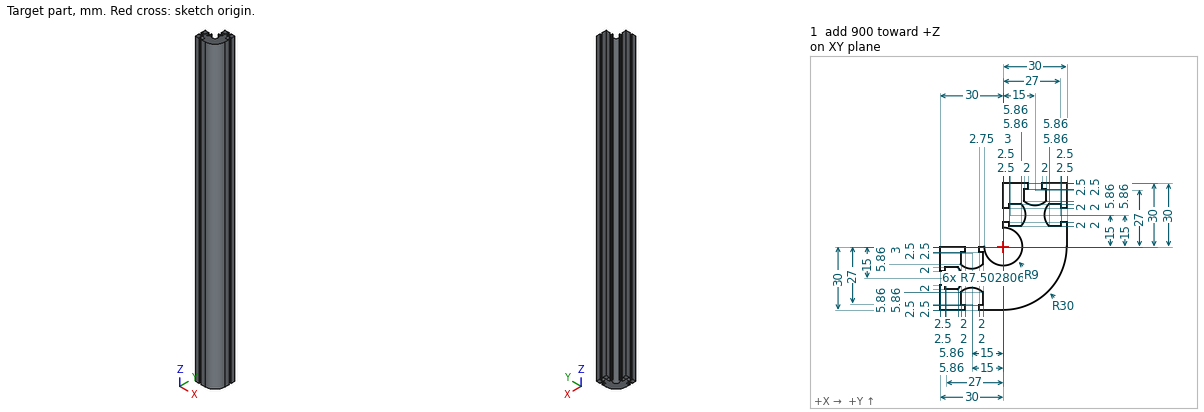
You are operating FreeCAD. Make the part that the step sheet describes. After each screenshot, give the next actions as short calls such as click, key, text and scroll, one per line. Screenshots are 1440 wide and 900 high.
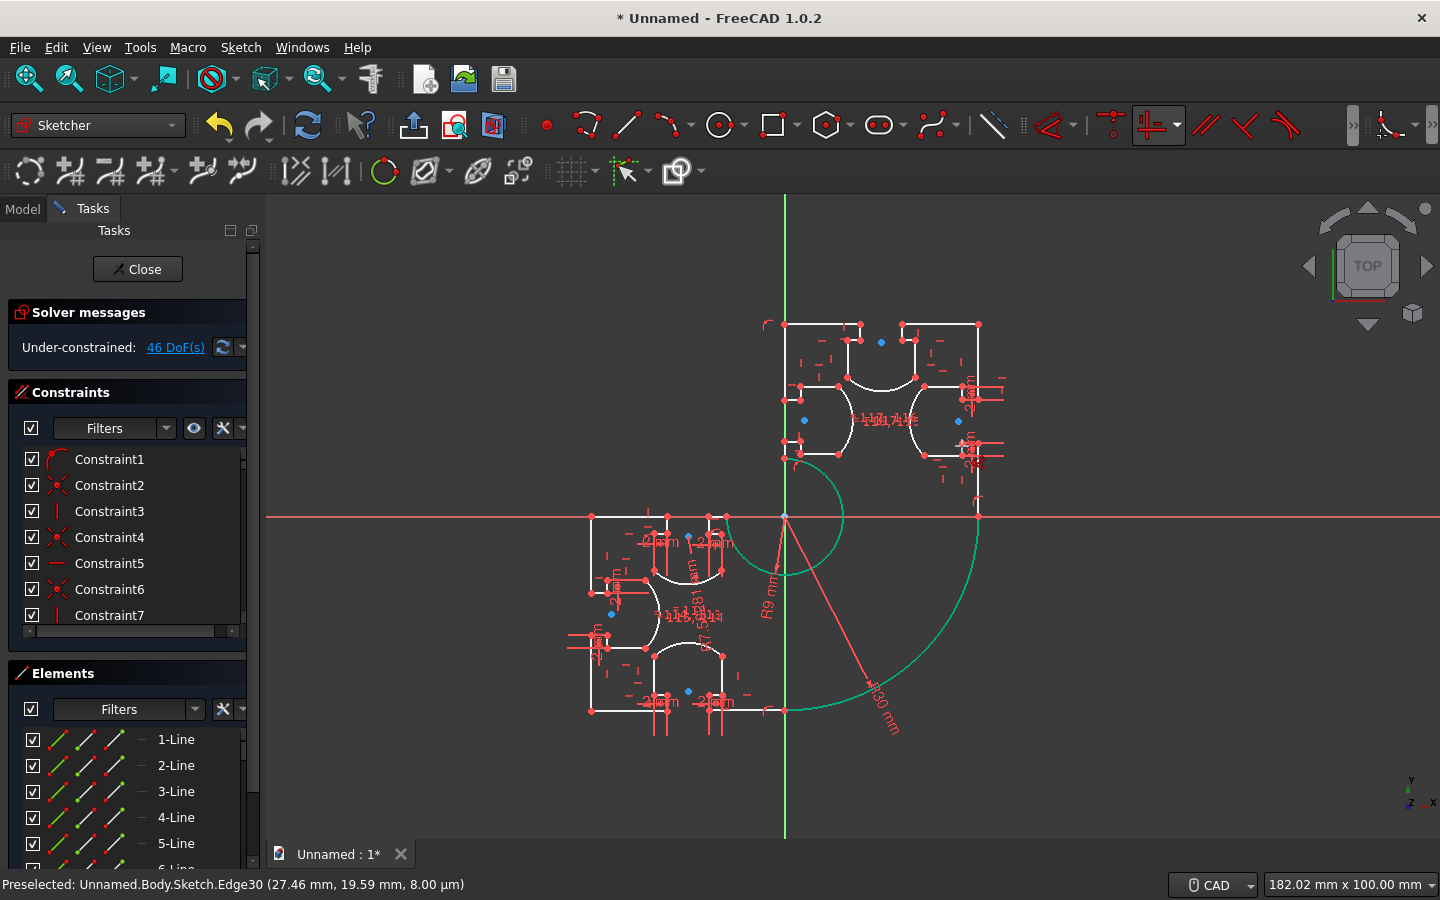
scroll(906, 340, up, 7)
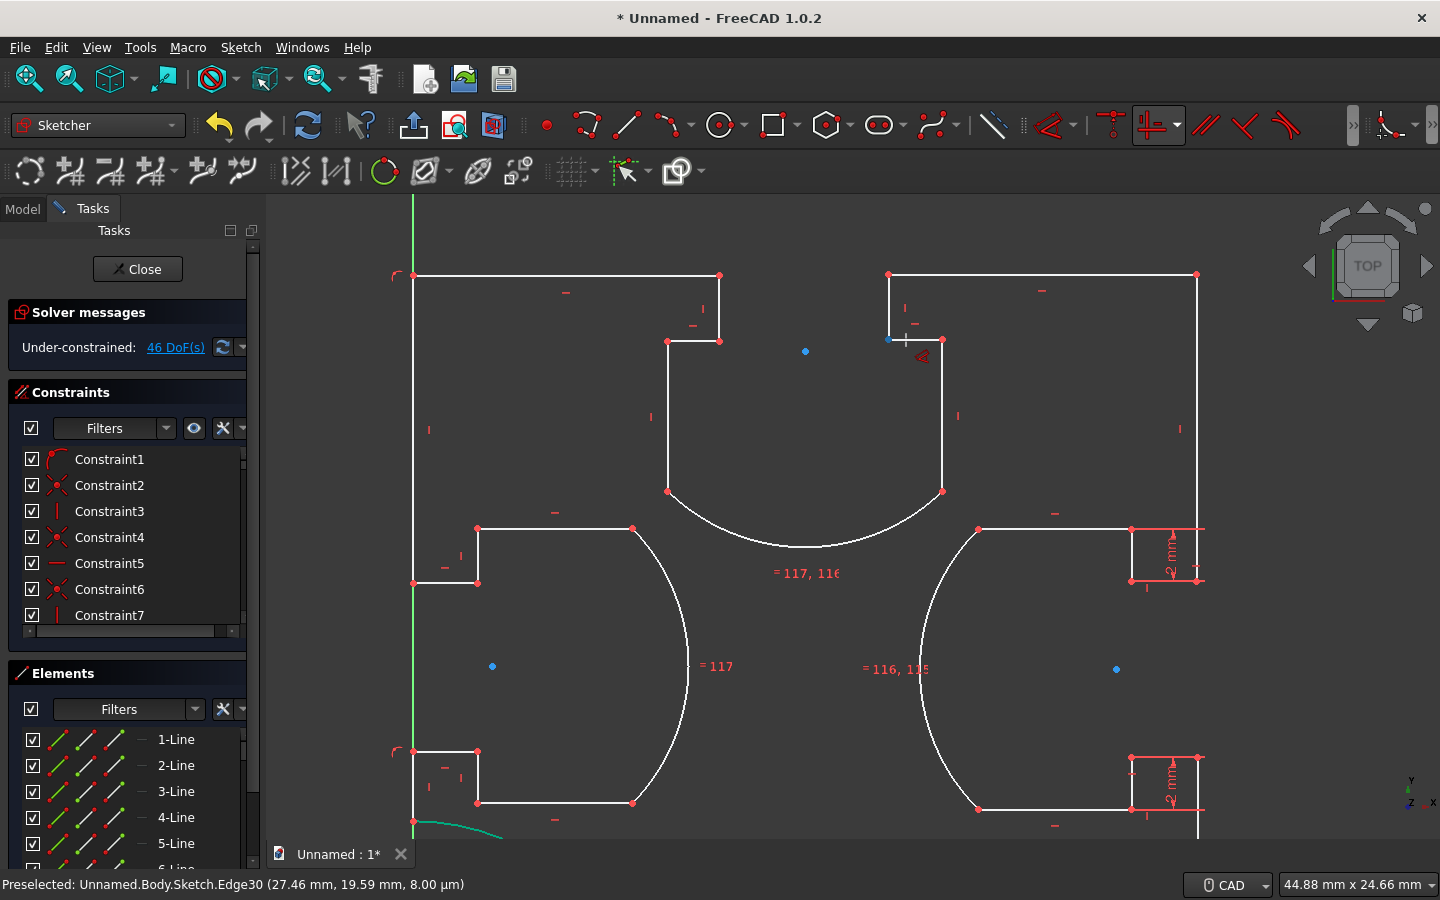
click(905, 340)
click(916, 306)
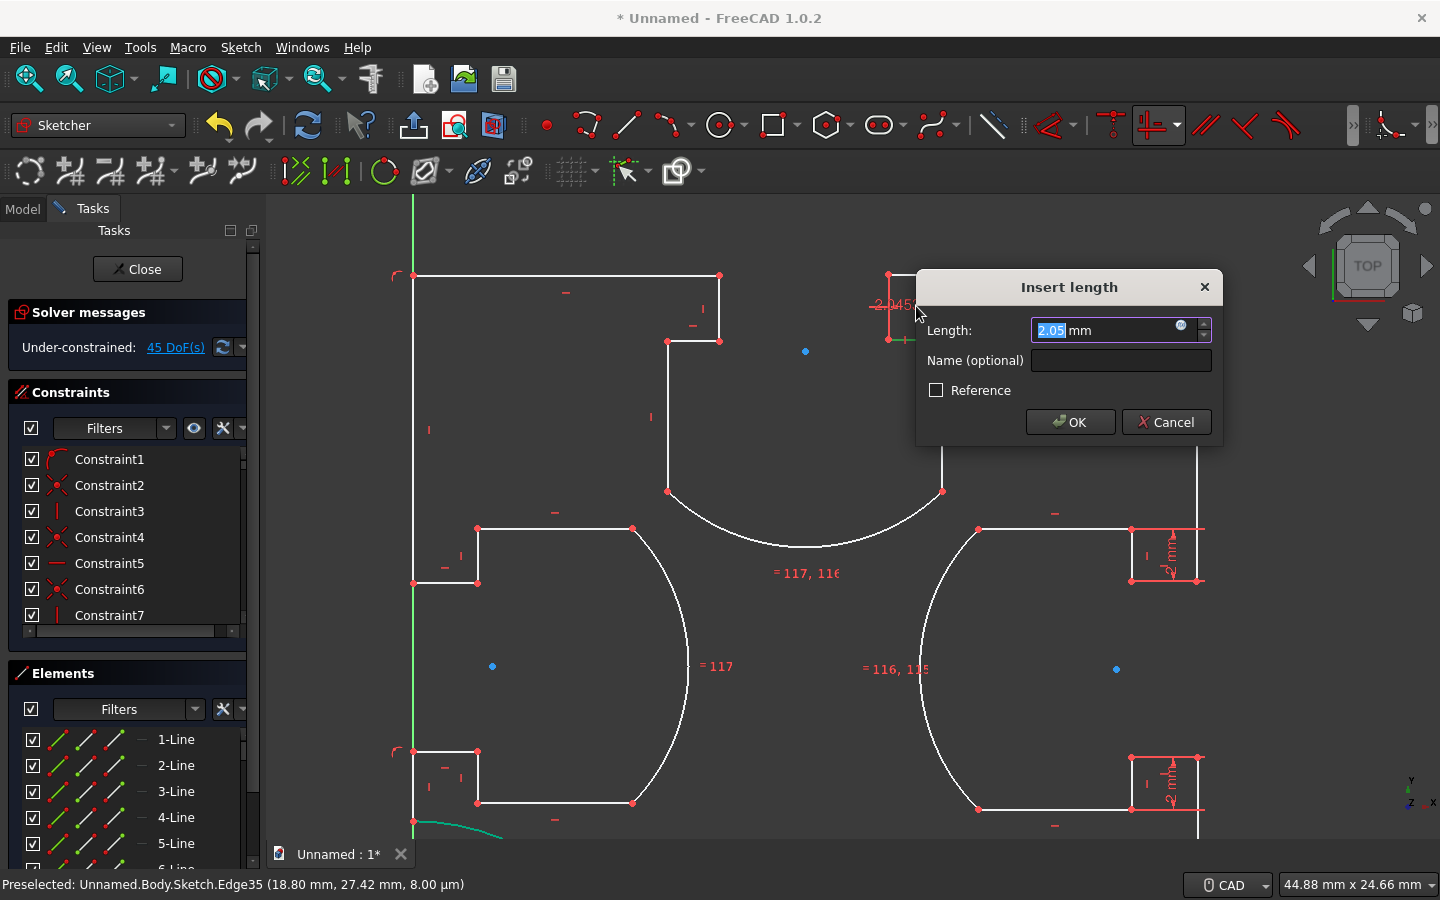
text(2)
key(Return)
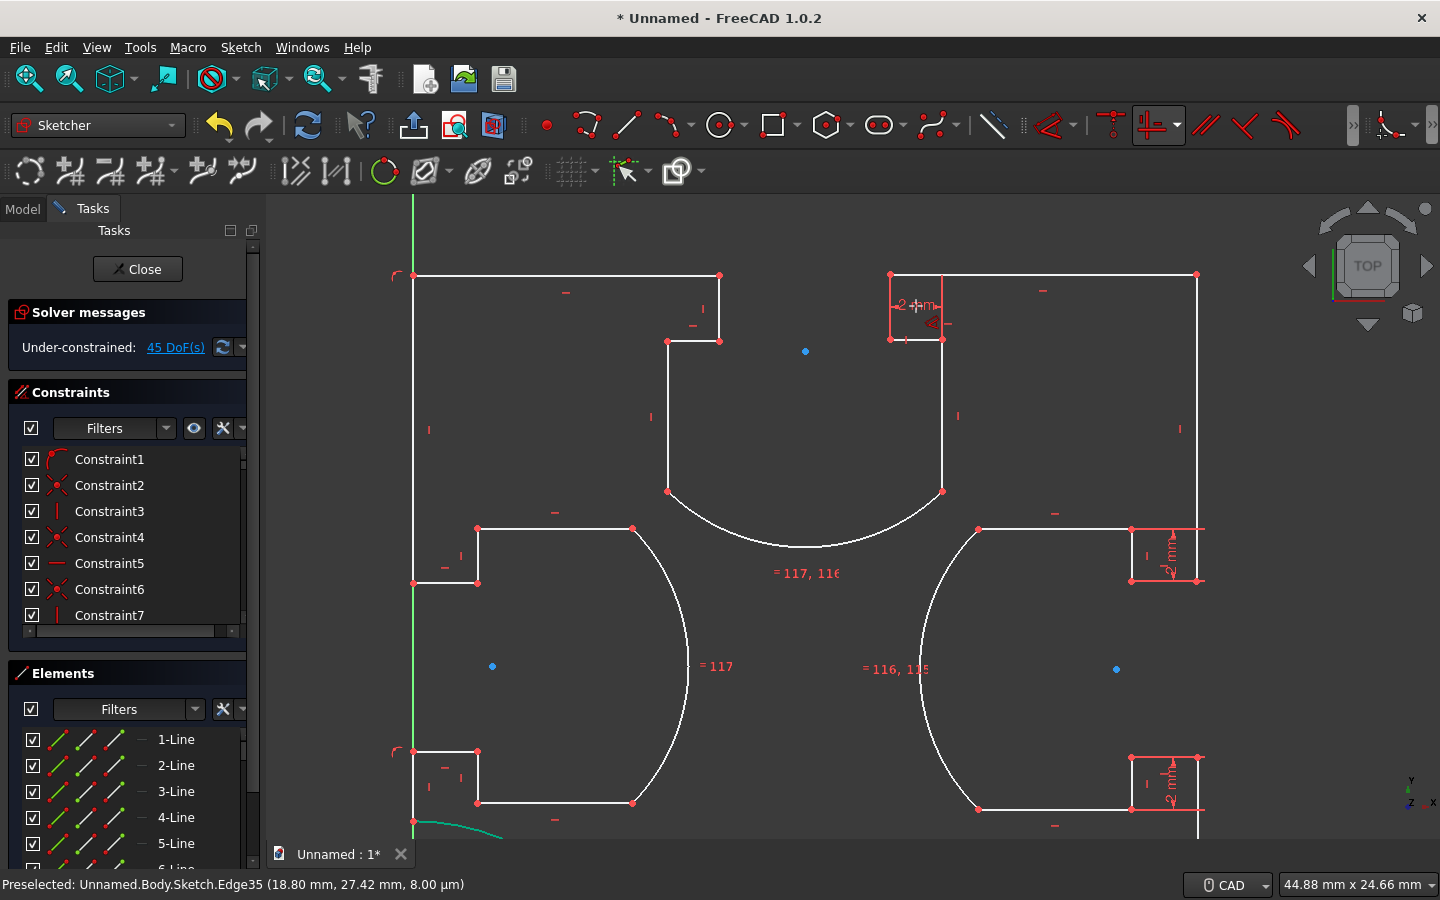
click(683, 341)
click(694, 307)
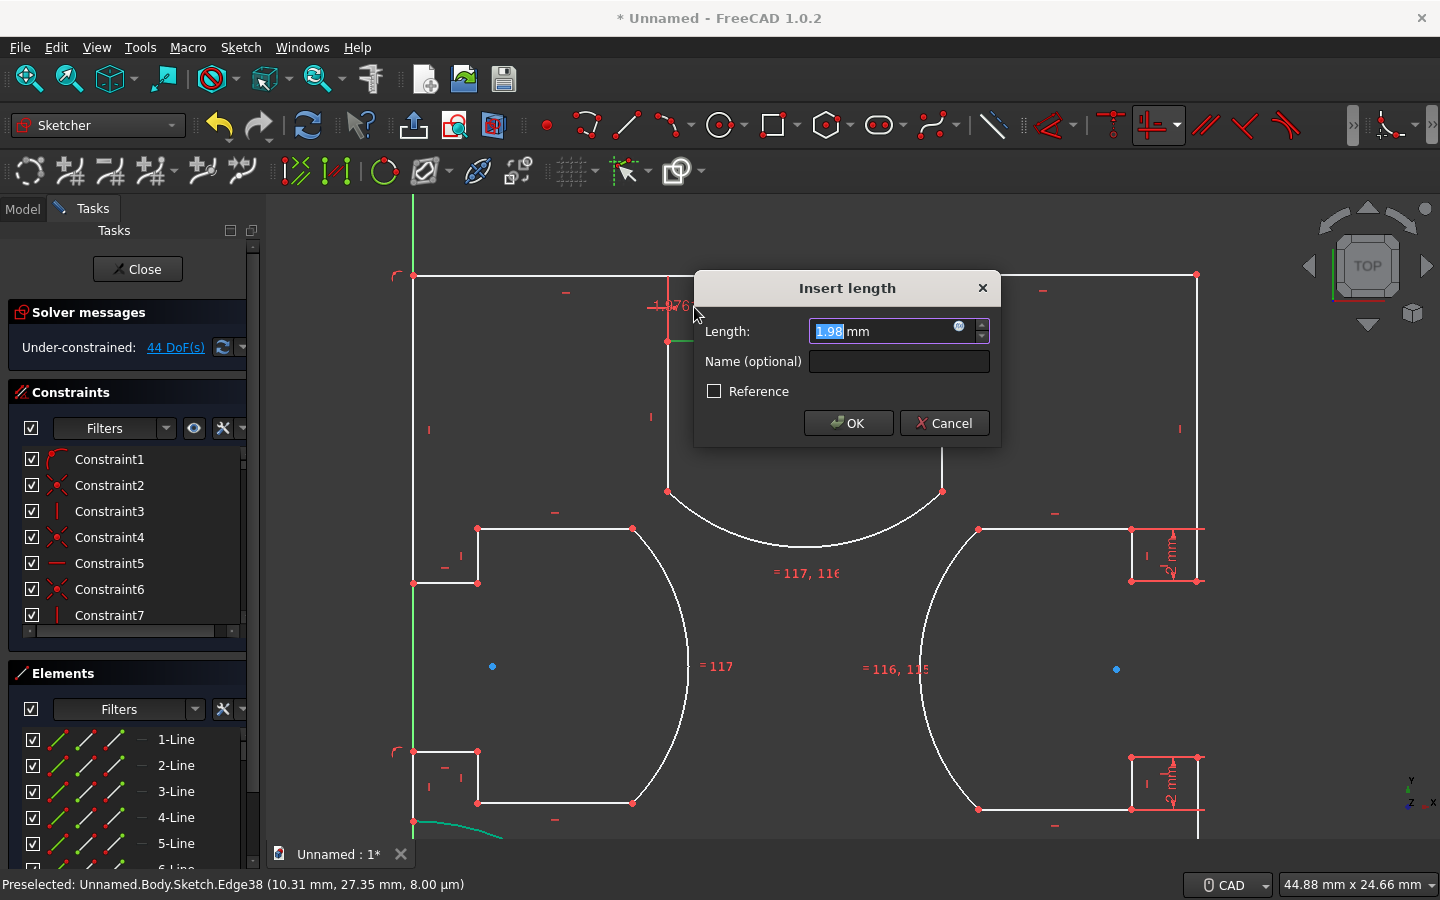
text(2)
key(Return)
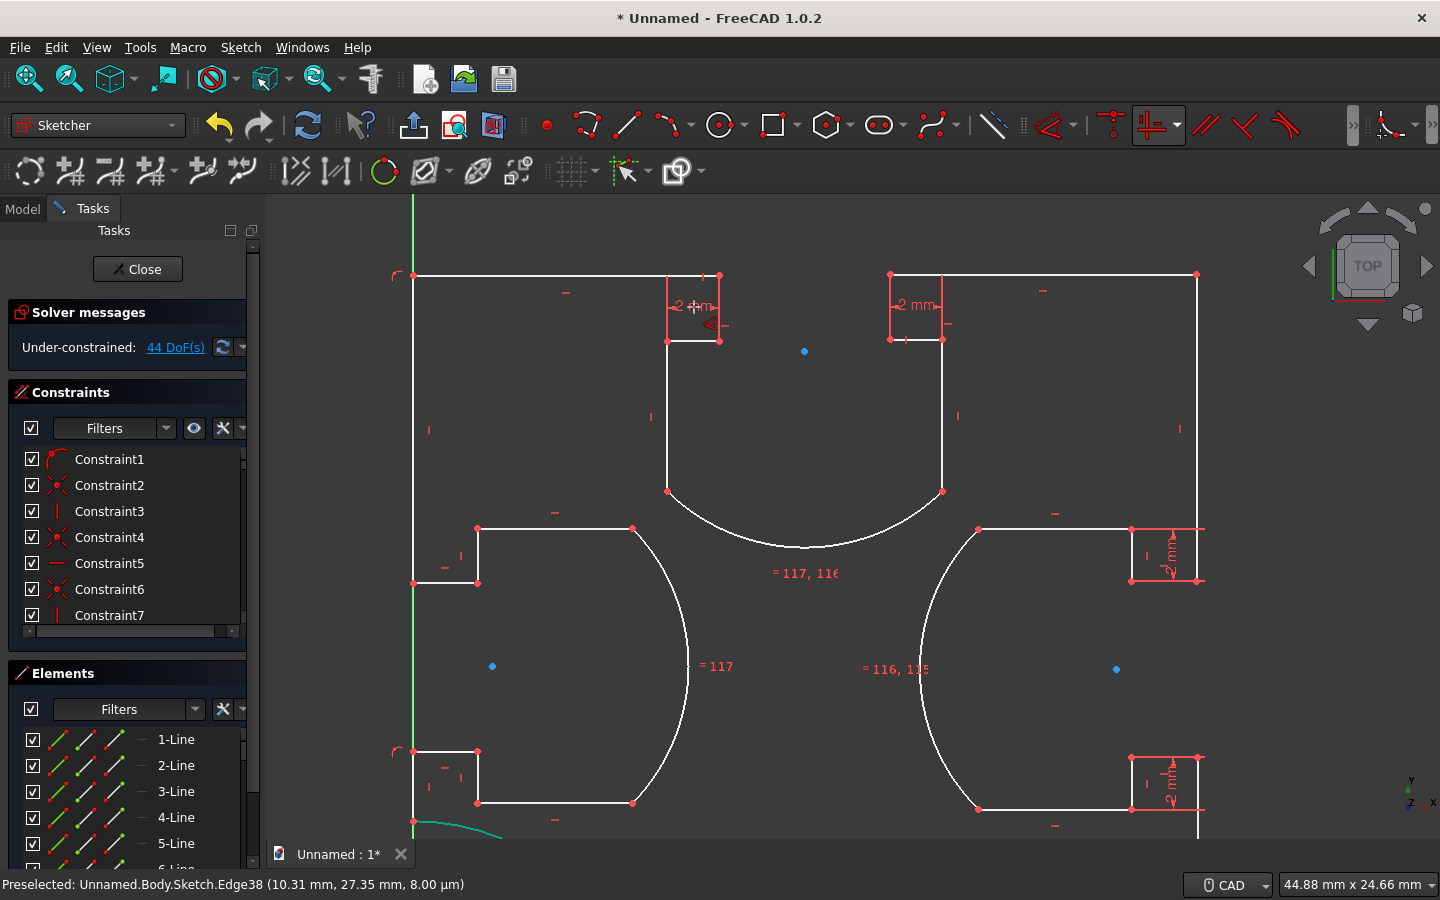
click(478, 567)
click(512, 556)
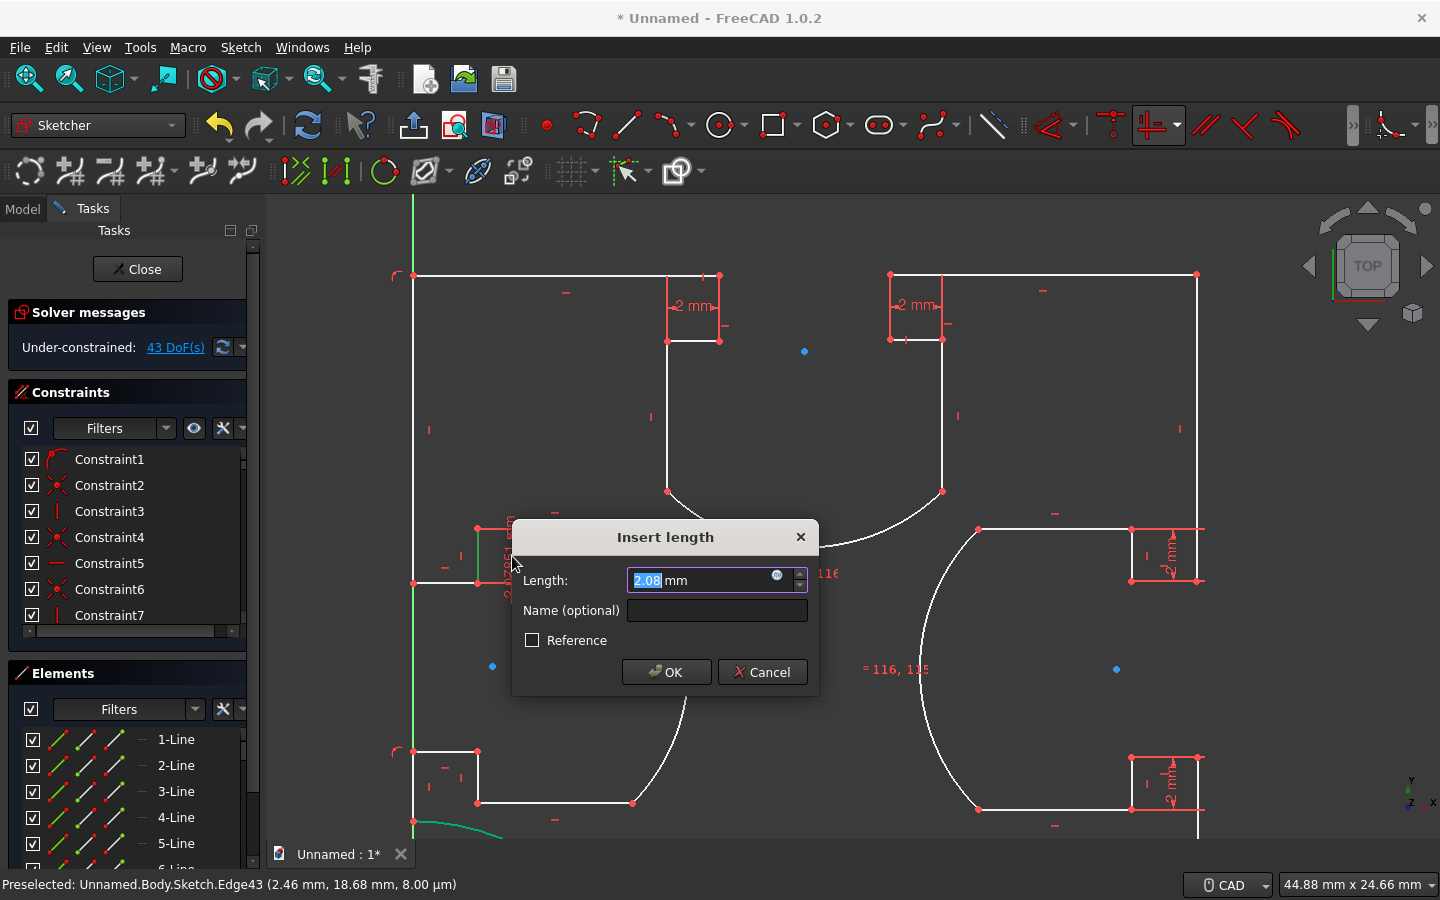
text(2)
key(Return)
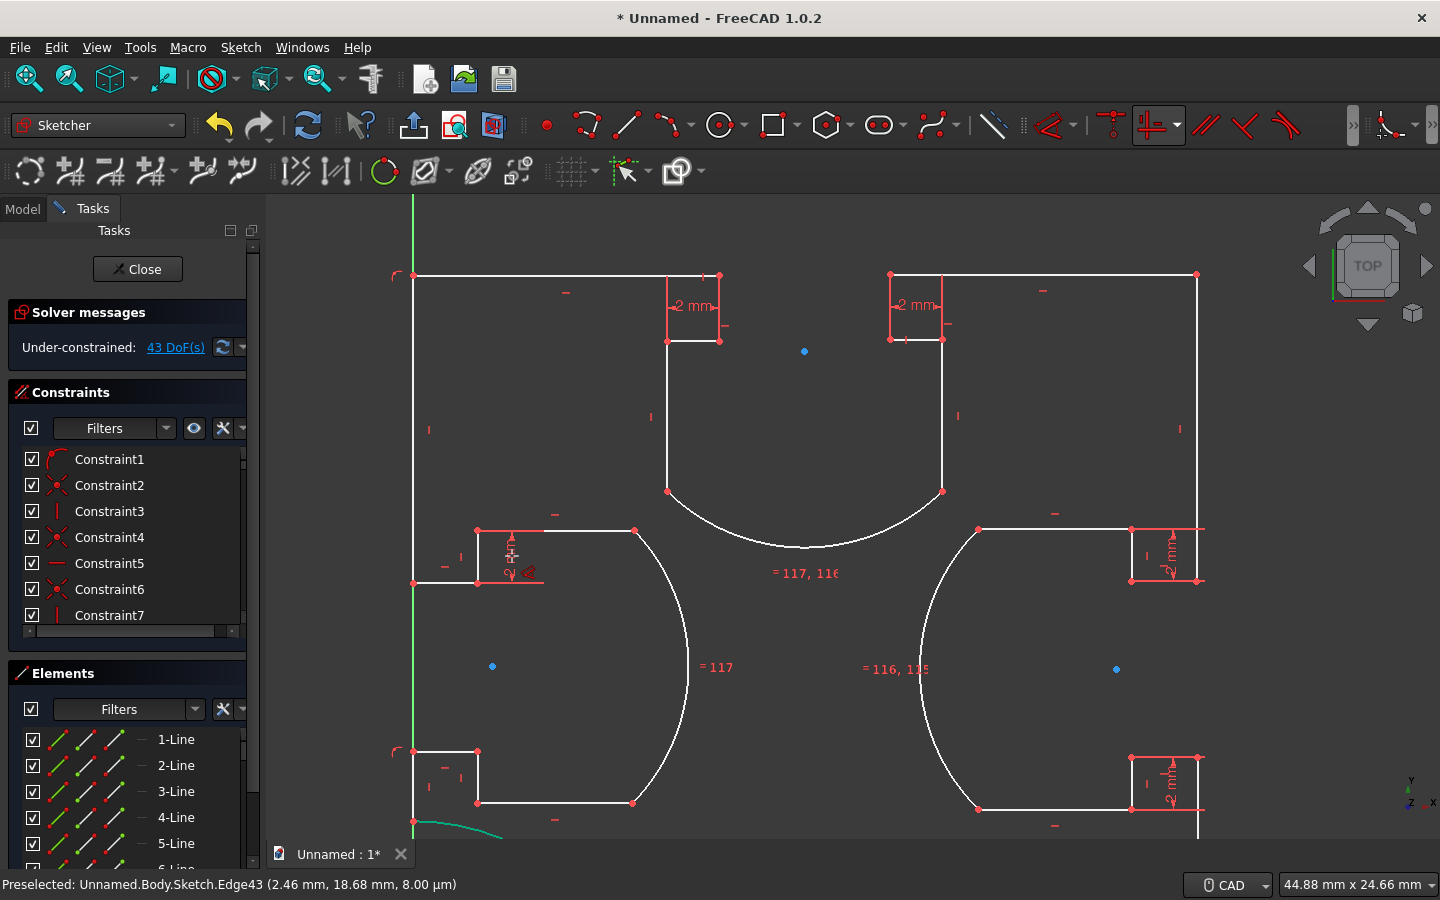
click(478, 788)
click(512, 778)